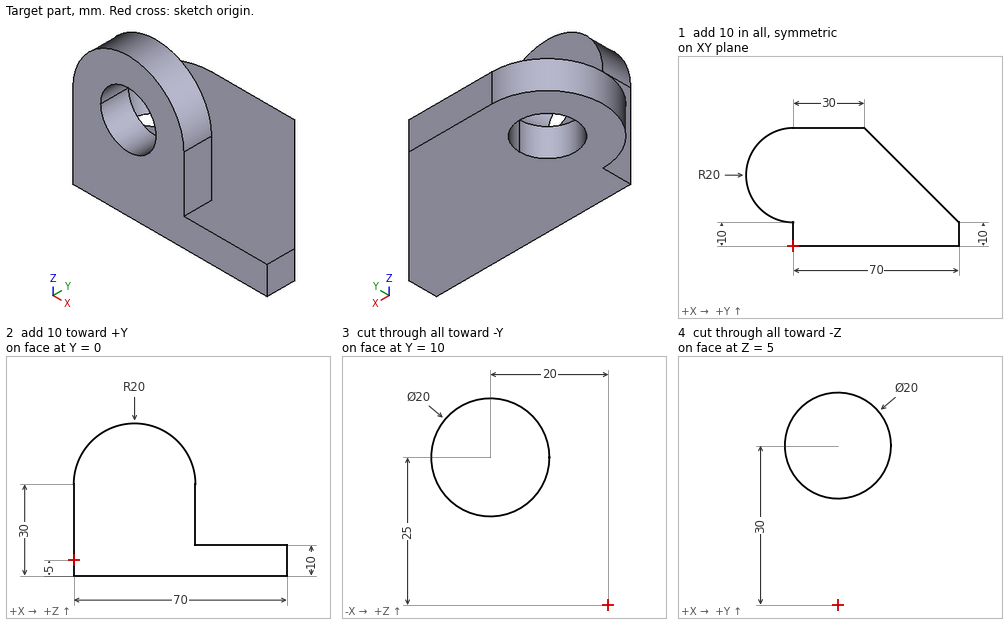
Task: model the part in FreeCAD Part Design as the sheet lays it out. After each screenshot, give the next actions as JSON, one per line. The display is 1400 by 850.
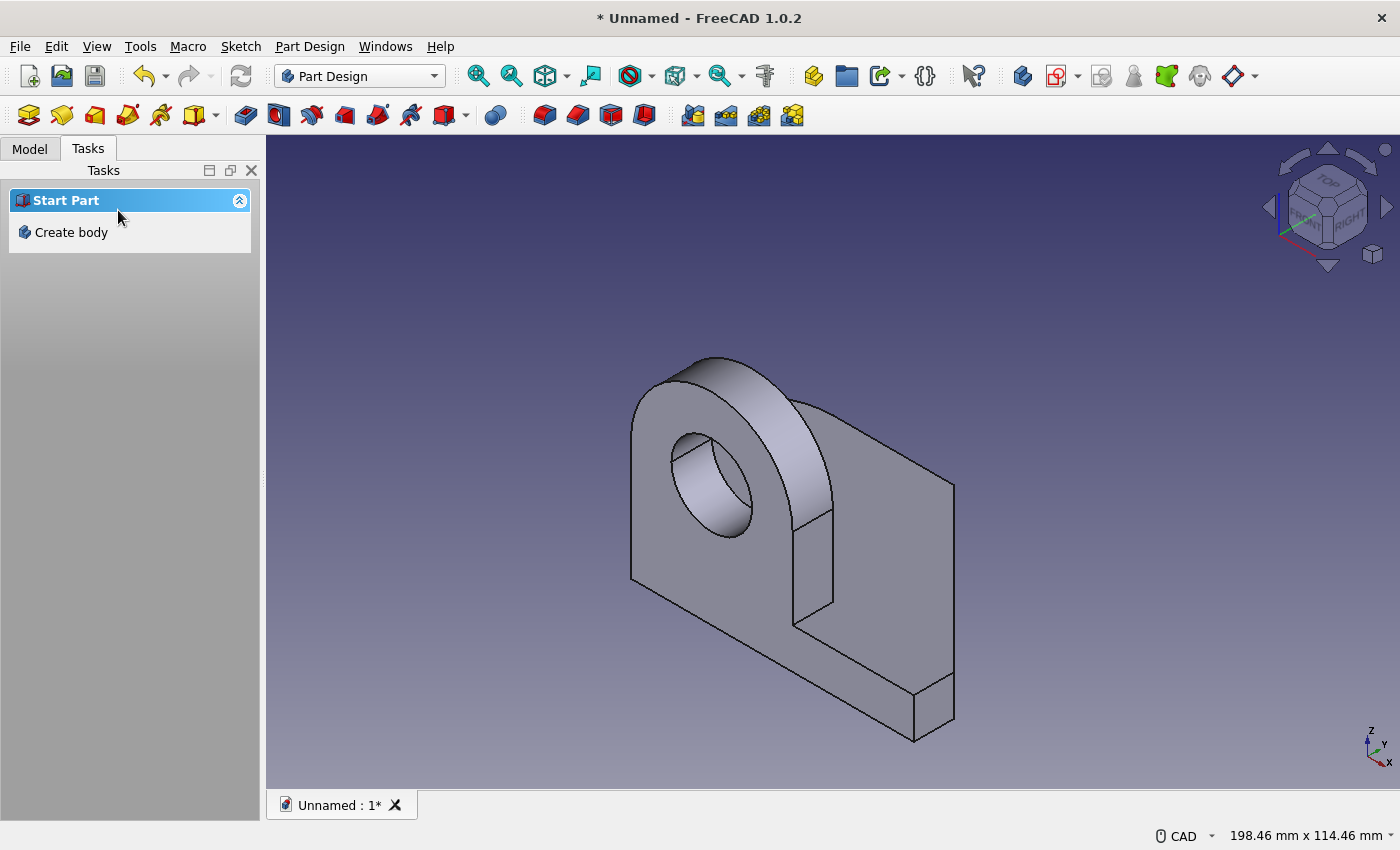
{"action": "left_click", "coordinate": [862, 514]}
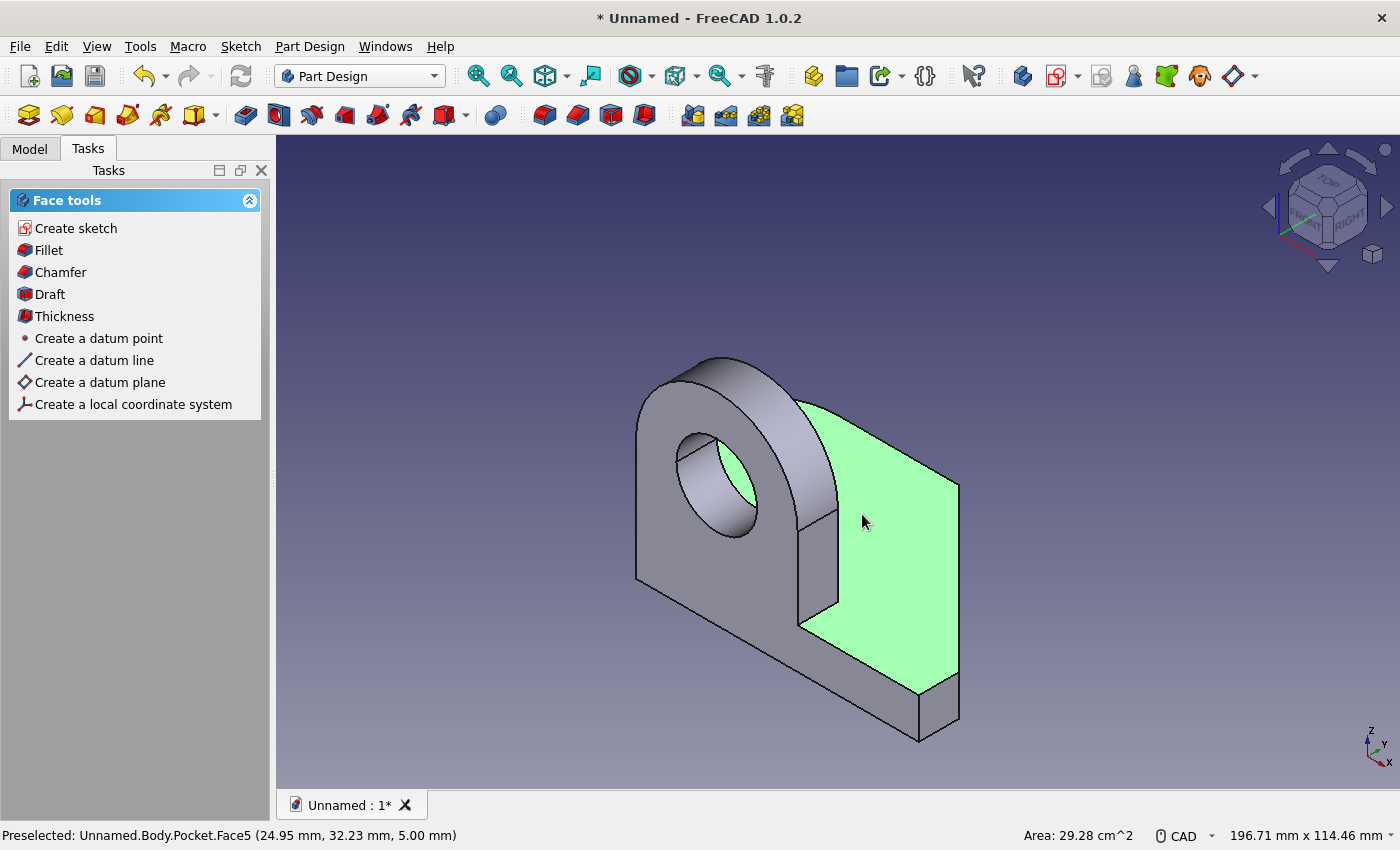
{"action": "left_click", "coordinate": [1056, 76]}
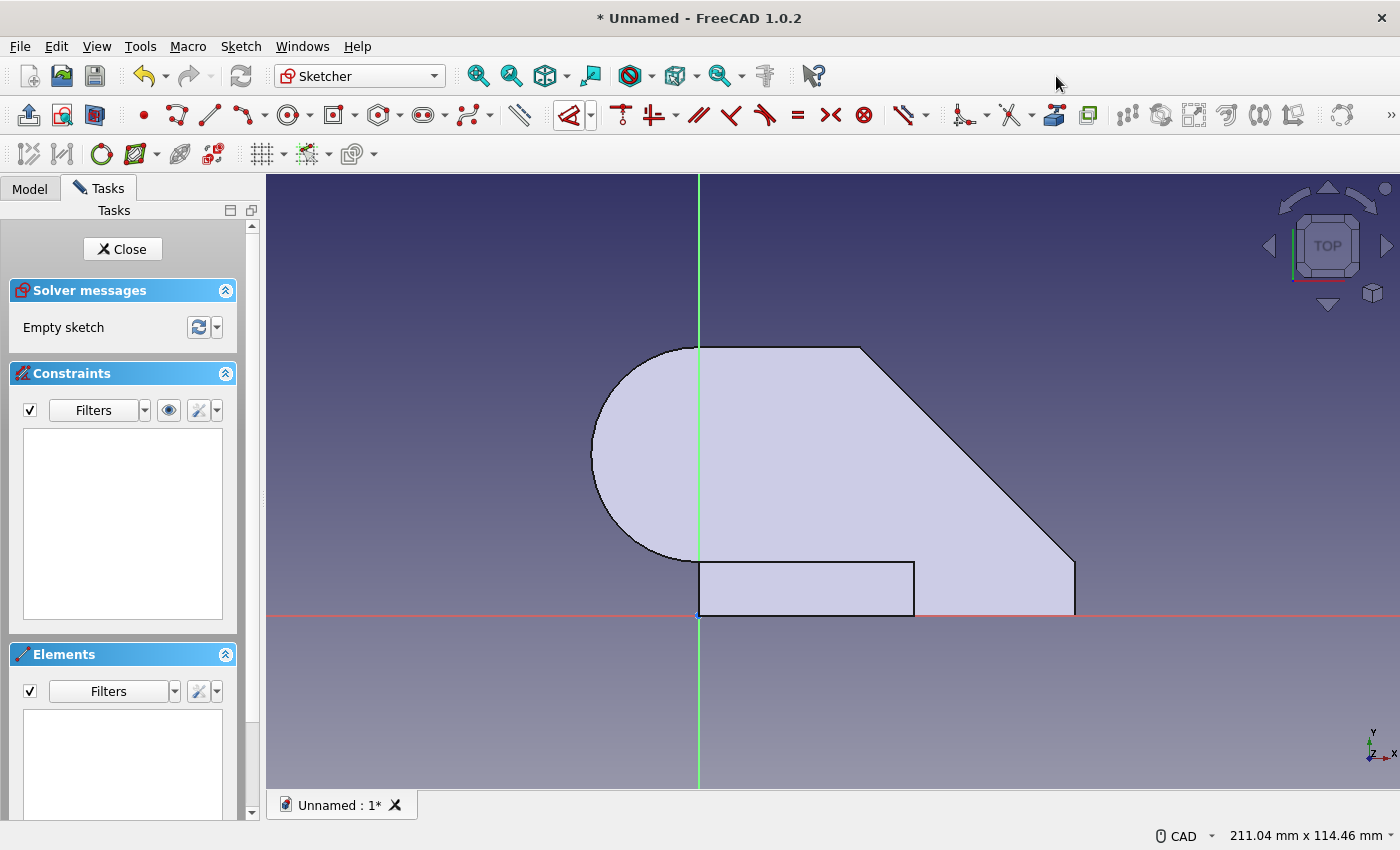
{"action": "scroll", "coordinate": [619, 541], "scroll_direction": "up", "scroll_amount": 3}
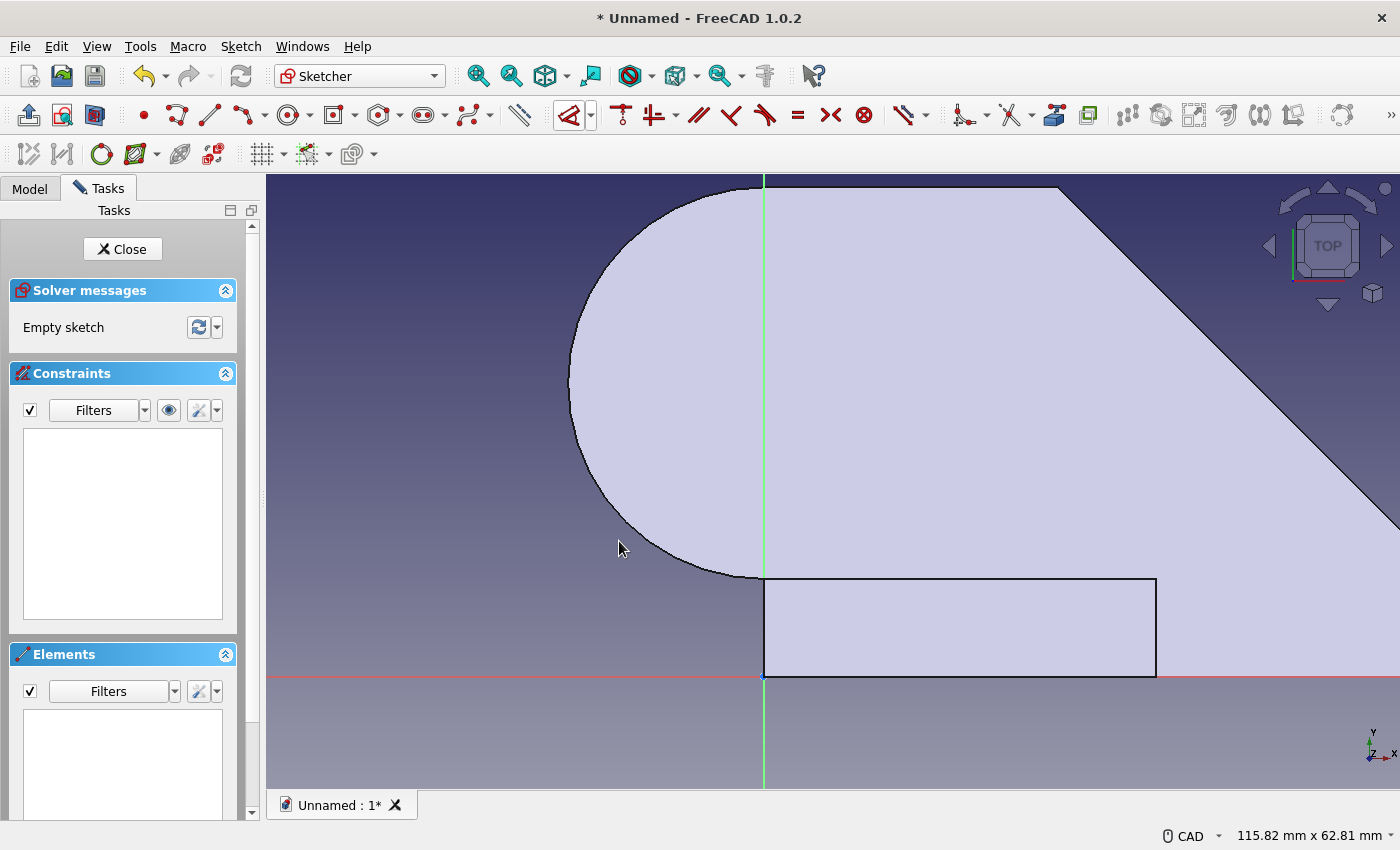
{"action": "left_click", "coordinate": [288, 116]}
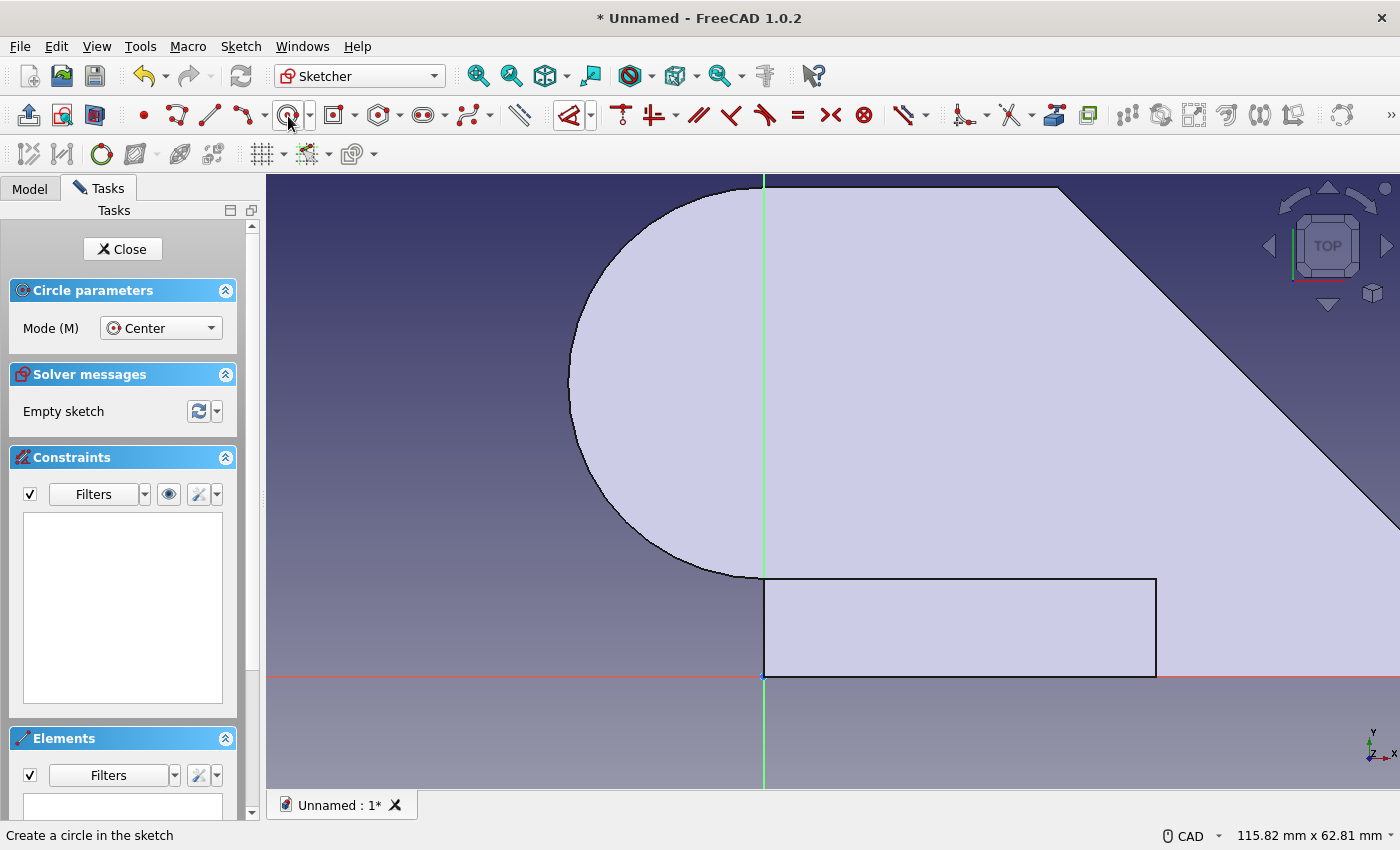
{"action": "left_click", "coordinate": [764, 383]}
{"action": "left_click", "coordinate": [833, 314]}
{"action": "key", "text": "Escape"}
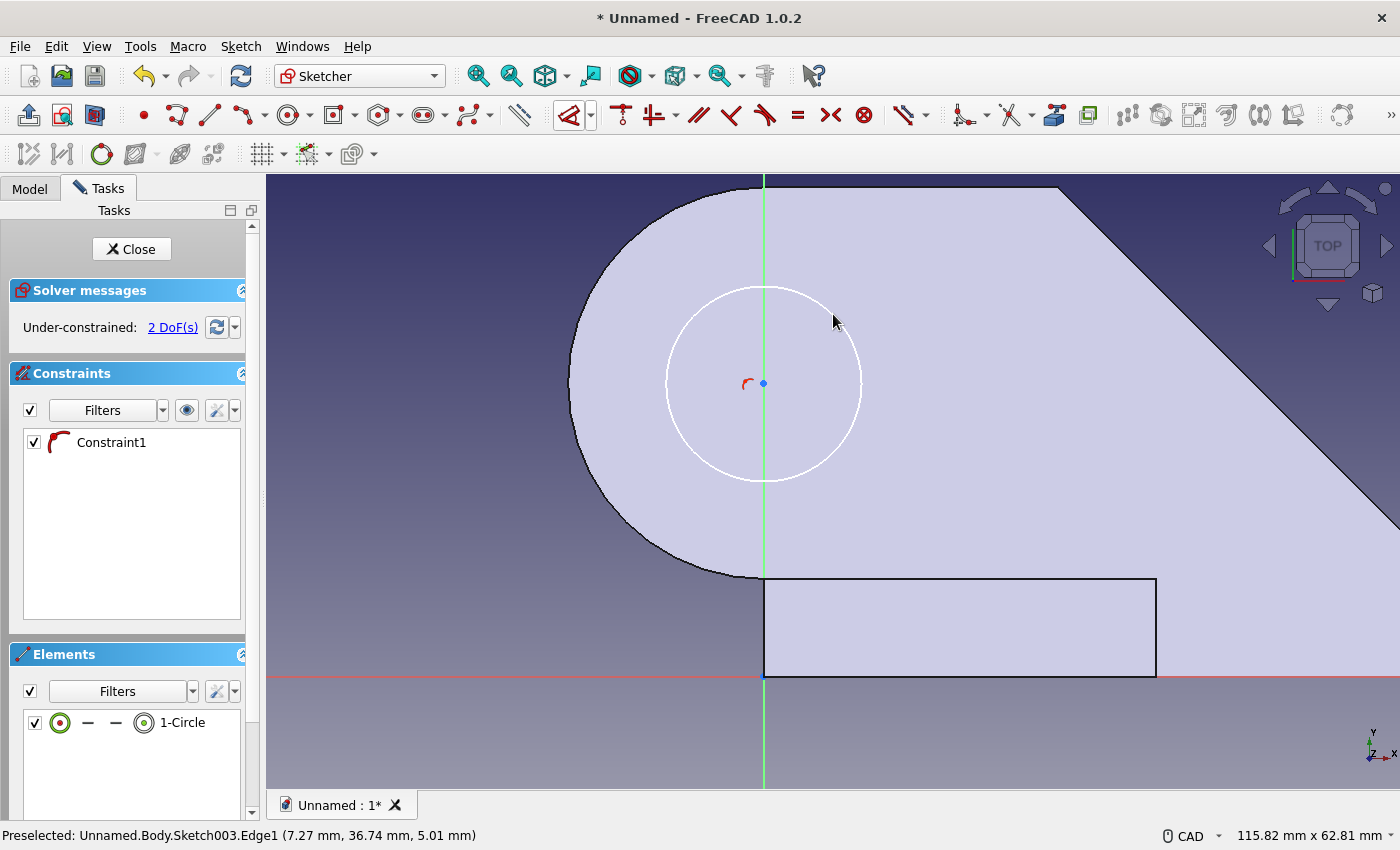
{"action": "left_click", "coordinate": [833, 315]}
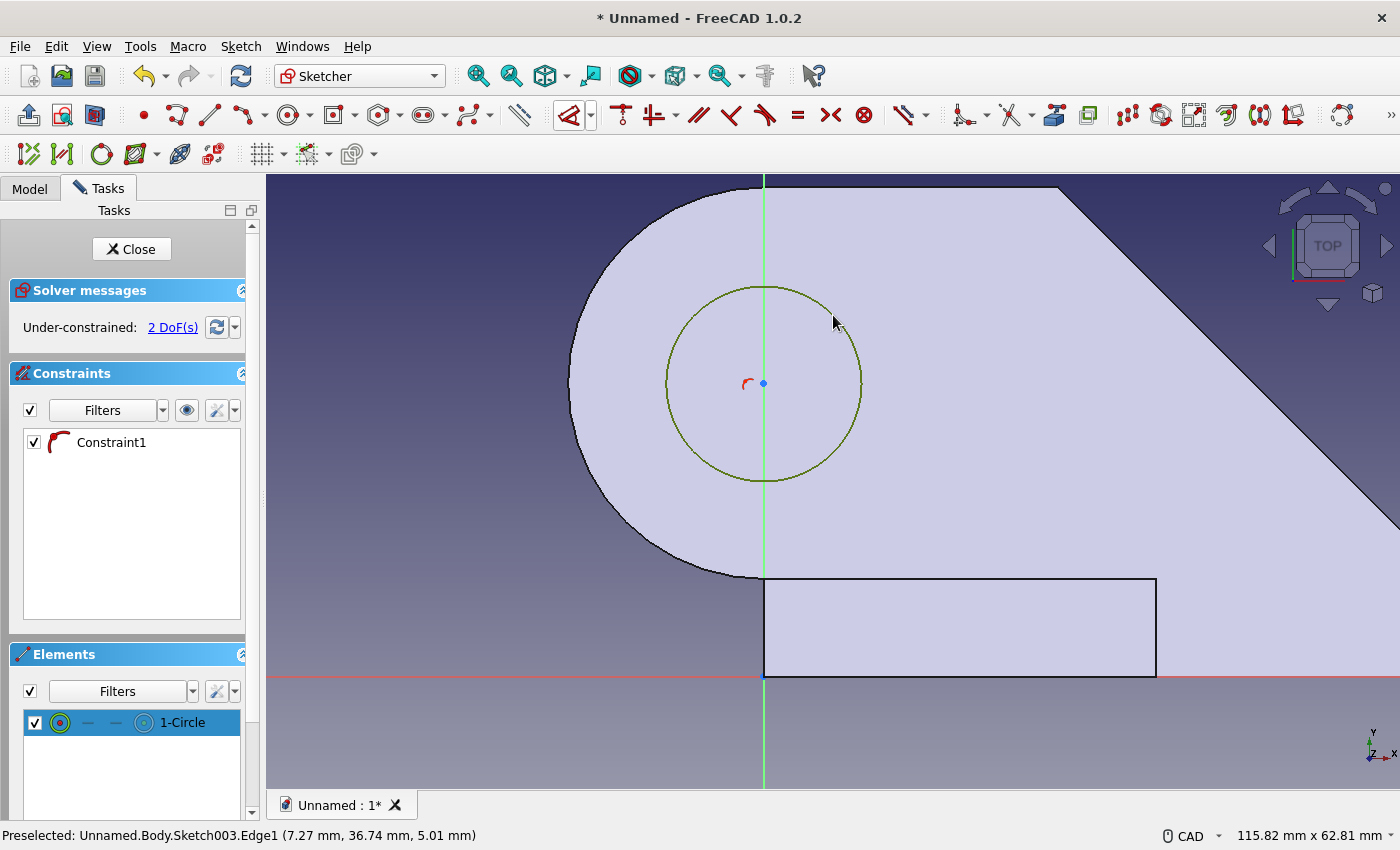
{"action": "key", "text": "k o"}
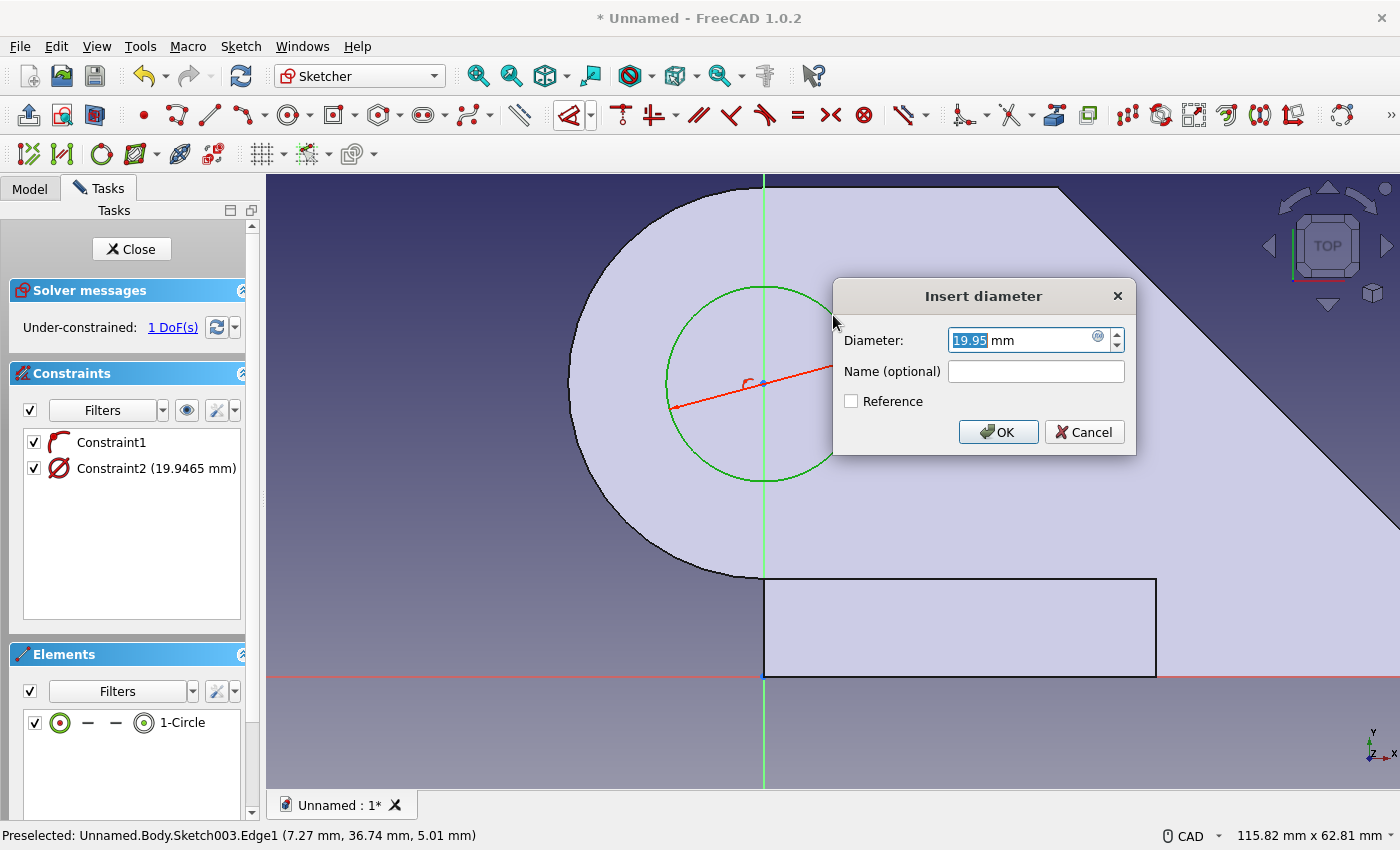
{"action": "type", "text": "20"}
{"action": "key", "text": "Return"}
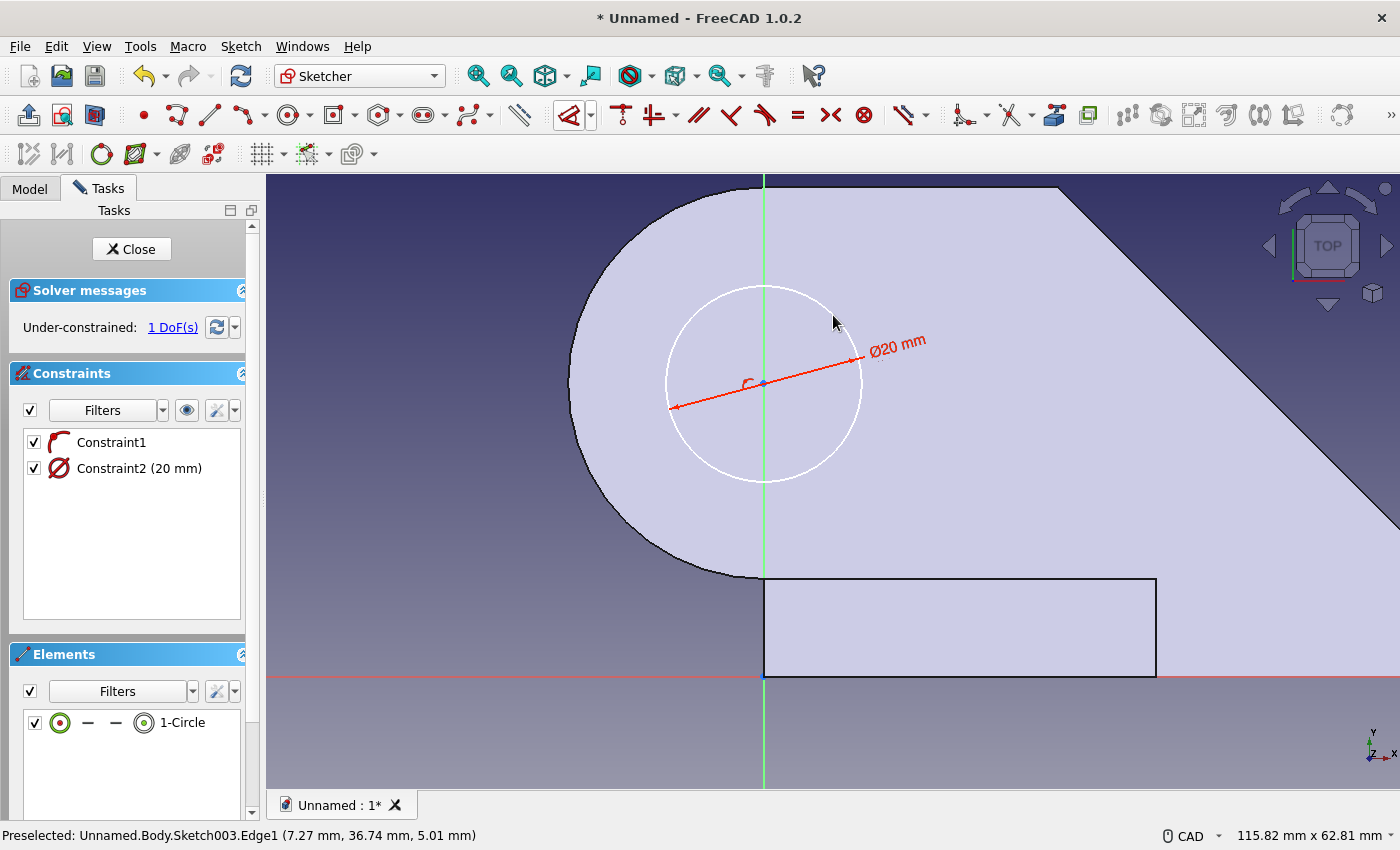
{"action": "left_click", "coordinate": [764, 384]}